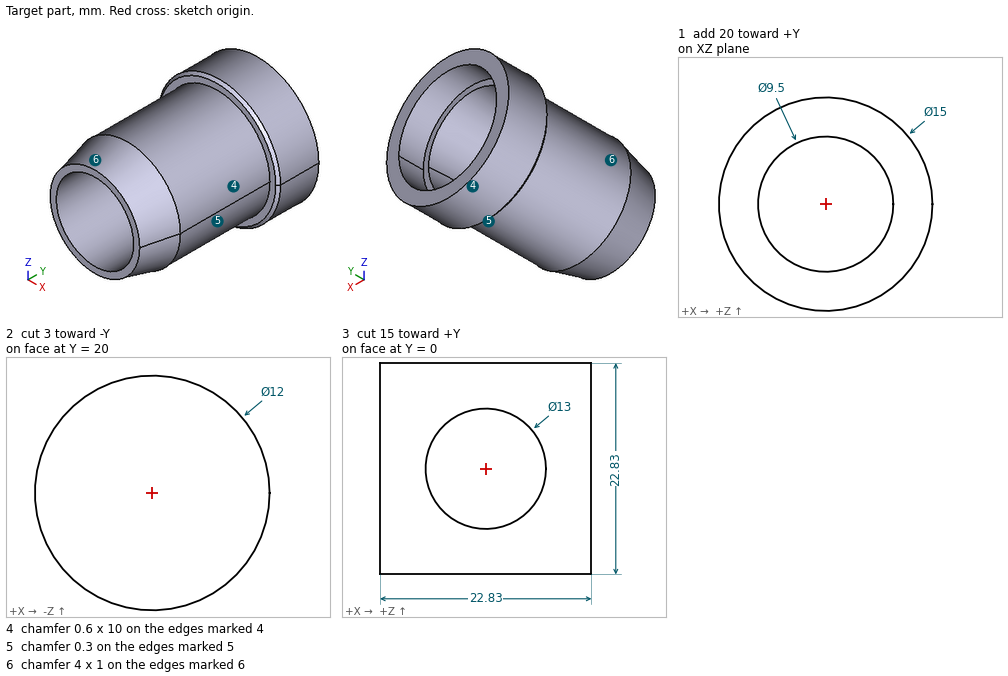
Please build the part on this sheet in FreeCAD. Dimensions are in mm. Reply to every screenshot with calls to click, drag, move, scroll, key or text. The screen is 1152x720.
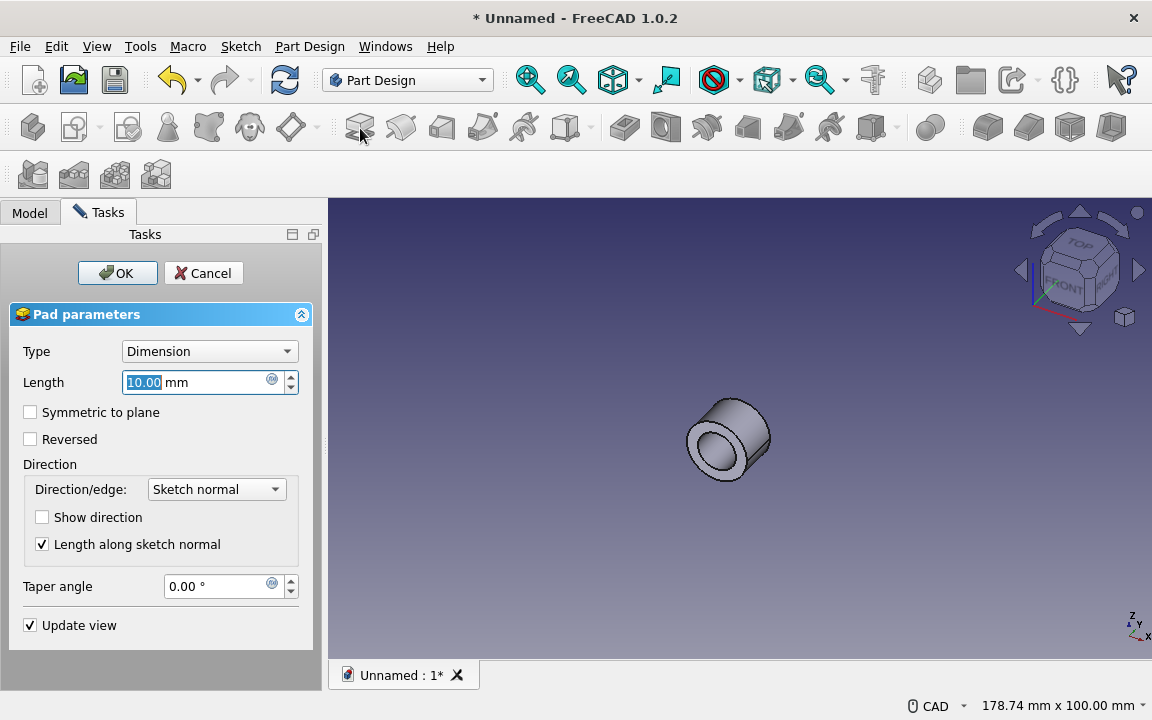
text(20)
key(Tab)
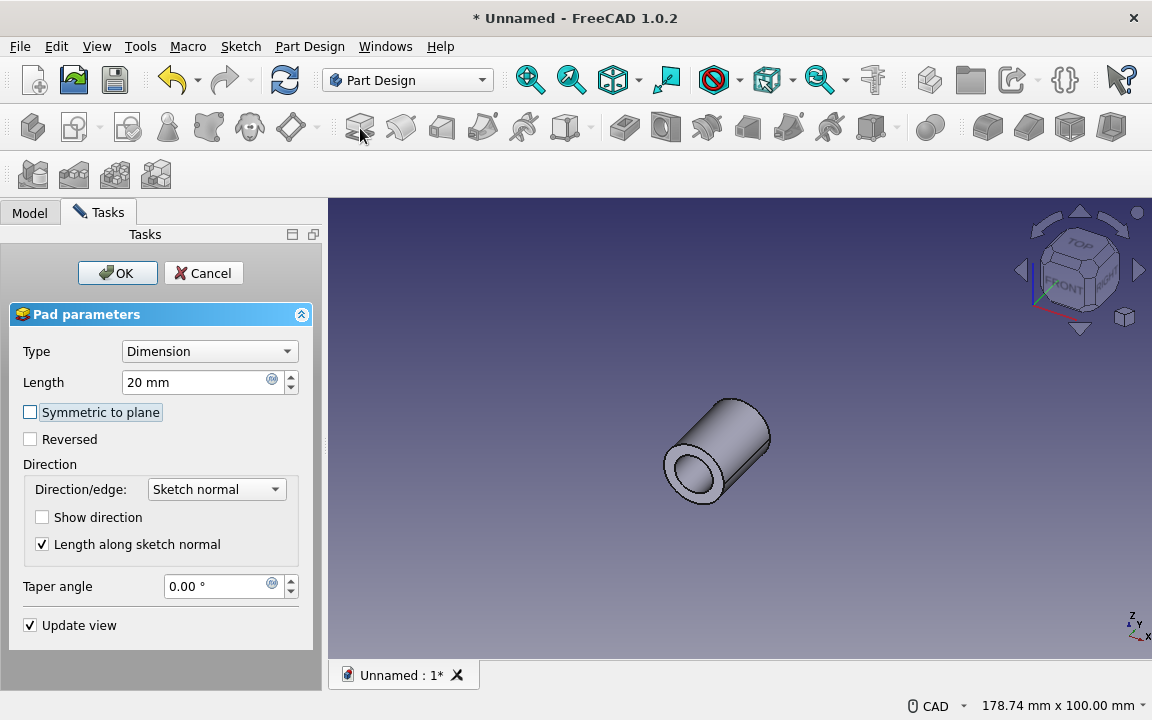
click(31, 439)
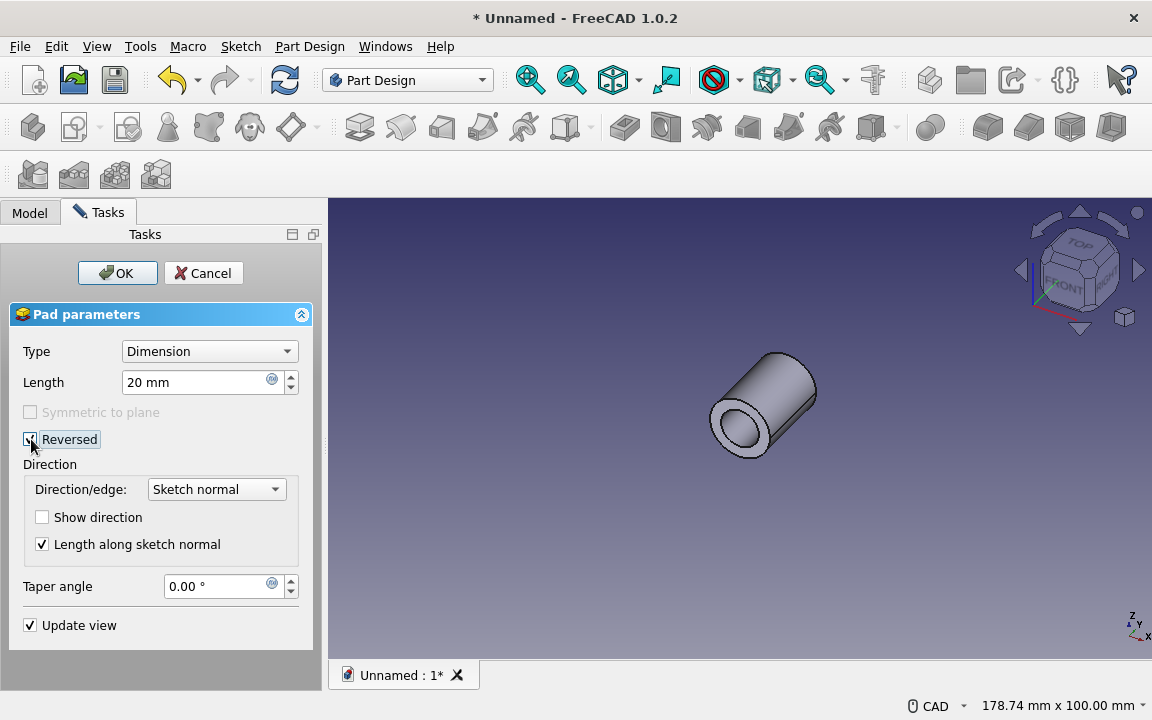
click(118, 273)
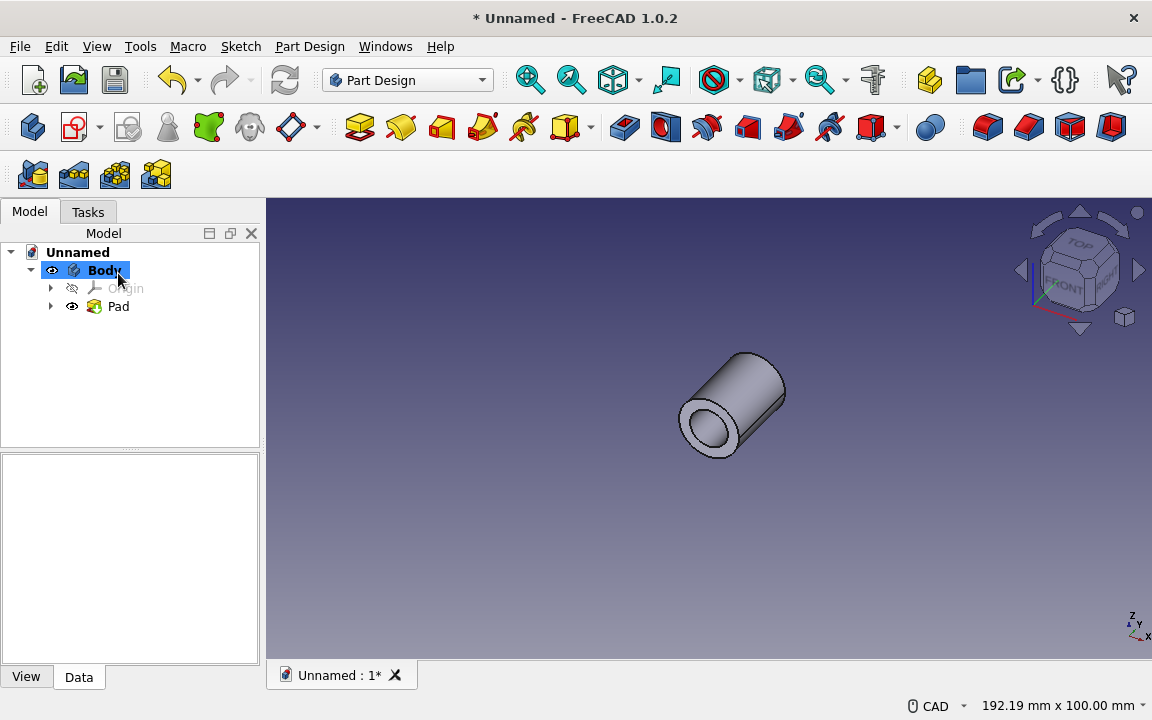
click(531, 80)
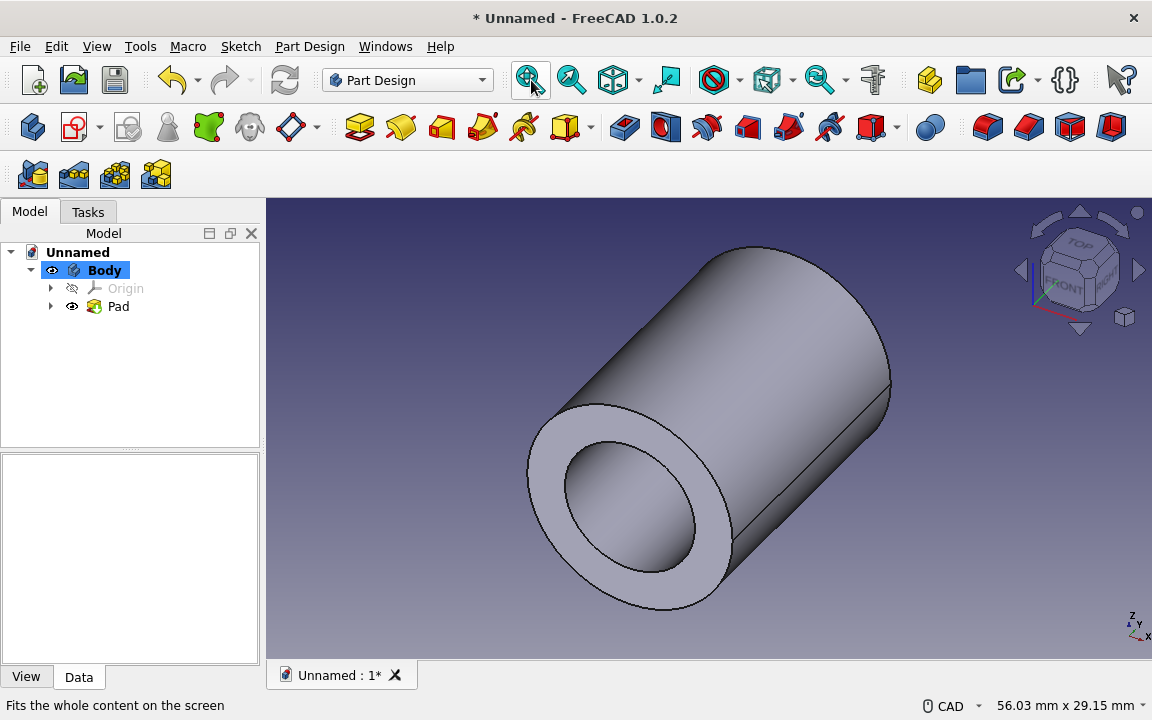
key(4)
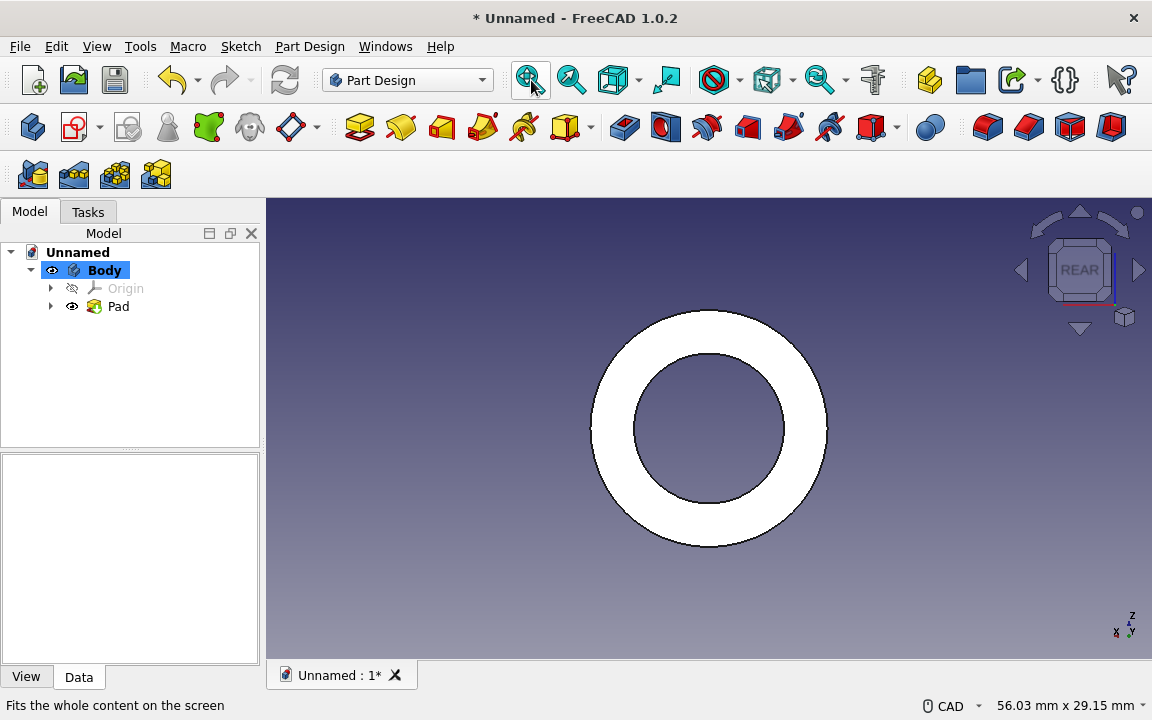
click(641, 360)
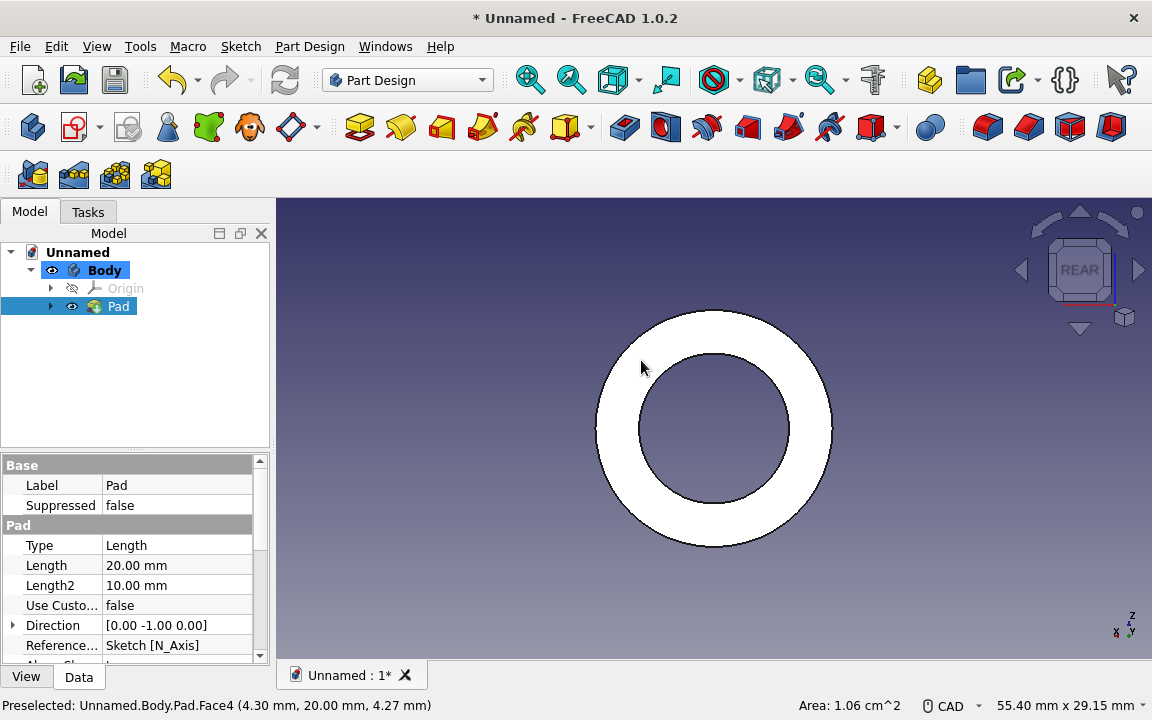
click(74, 128)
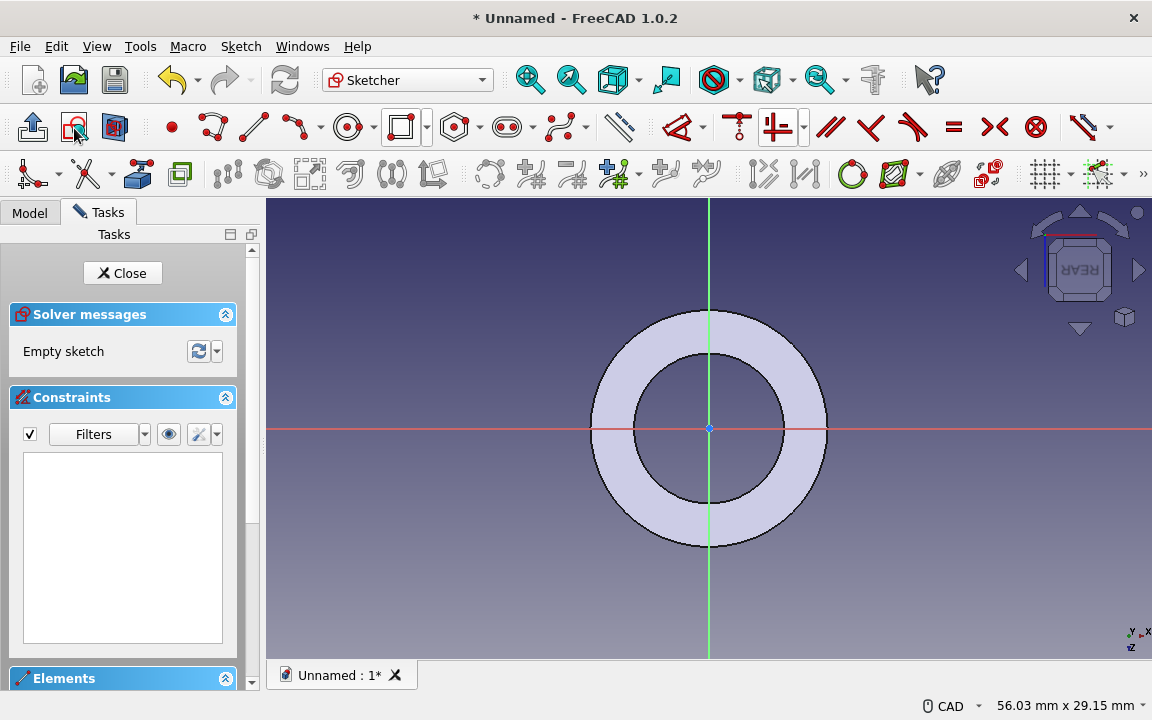
scroll(848, 428, up, 2)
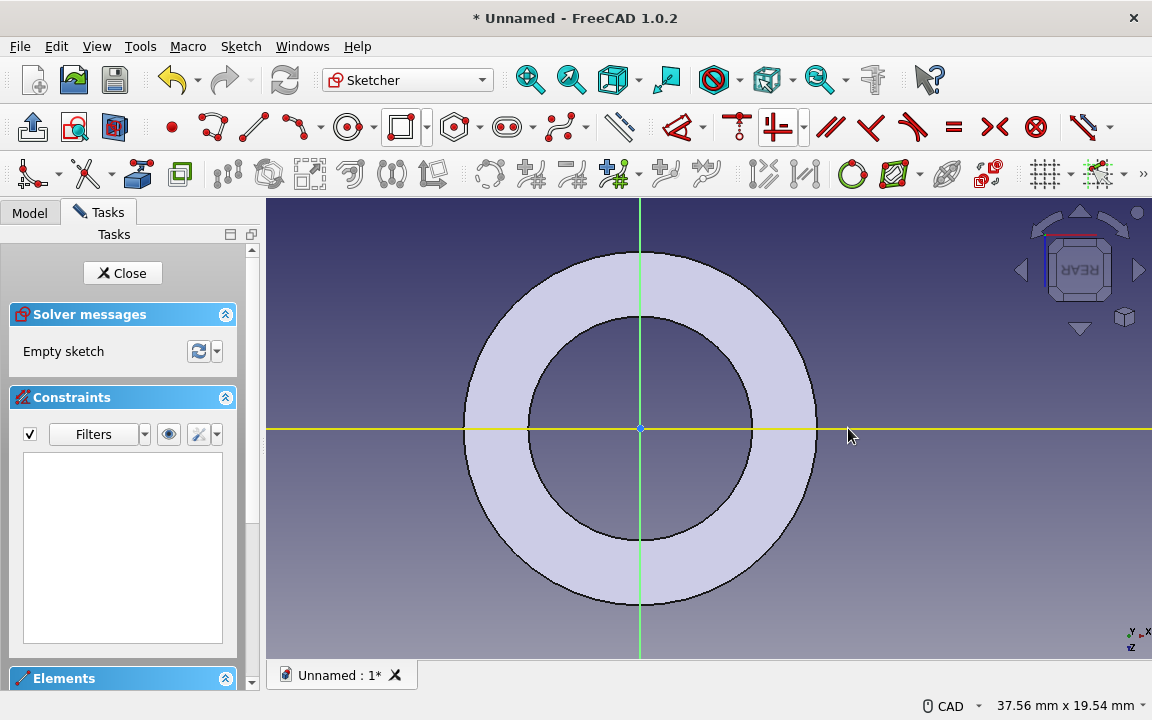
click(348, 128)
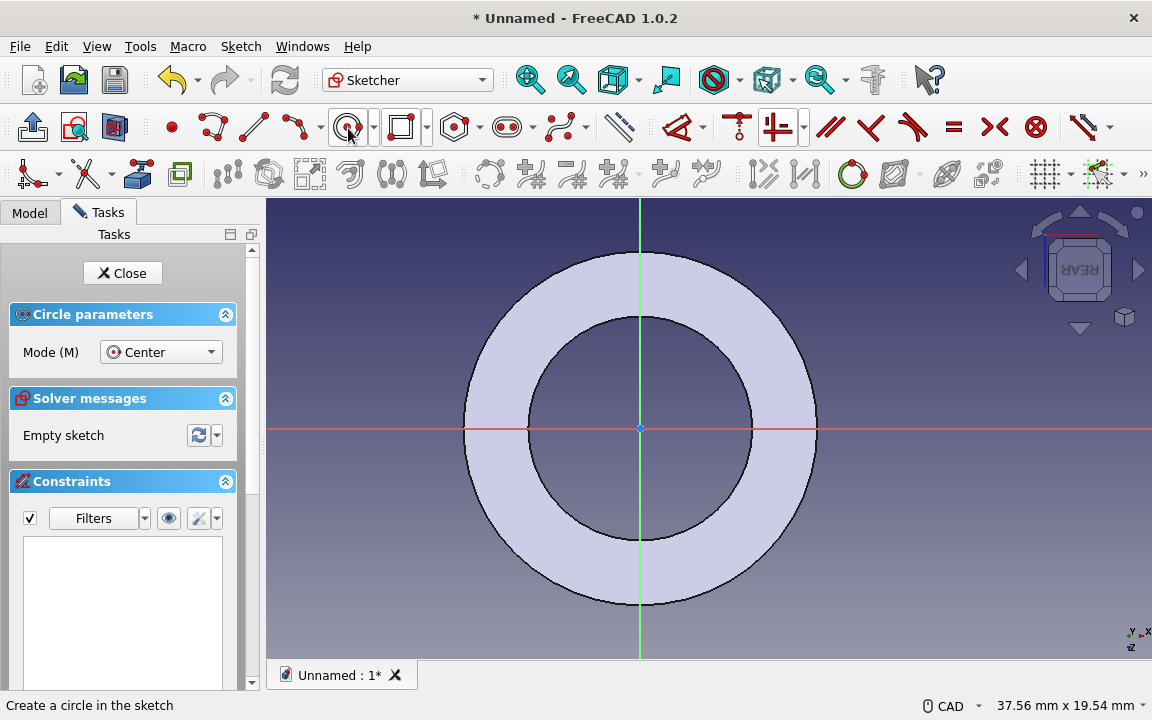
click(640, 428)
move(740, 328)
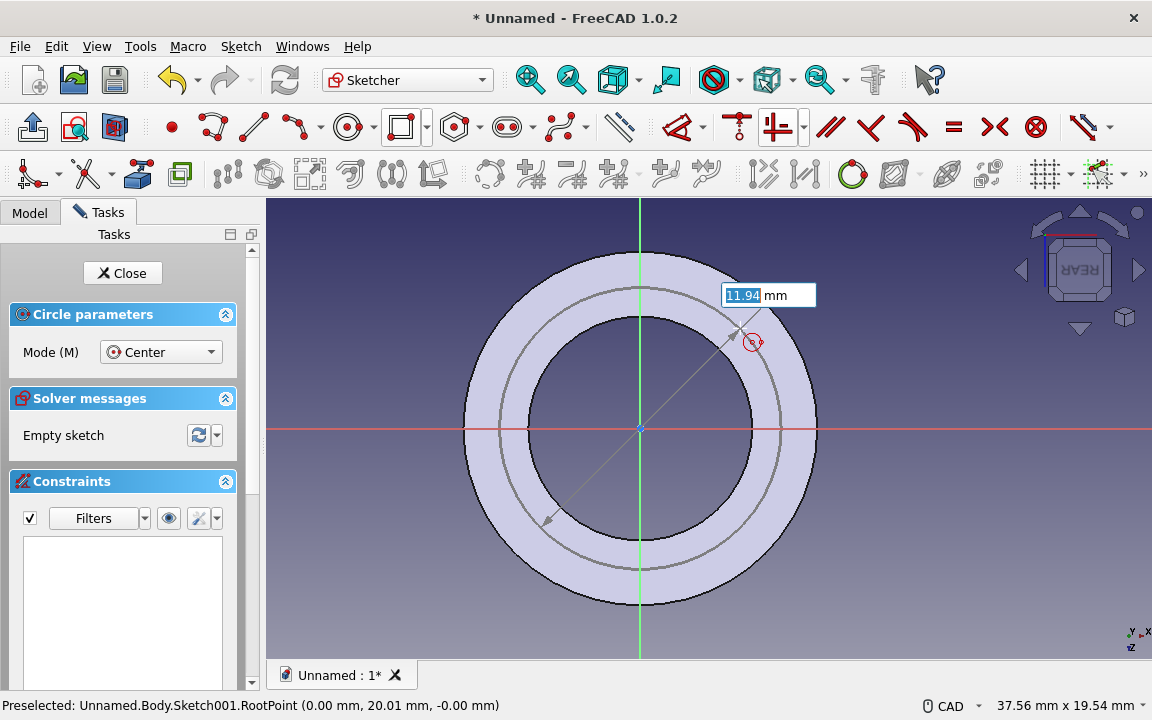
text(12)
key(Return)
key(Escape)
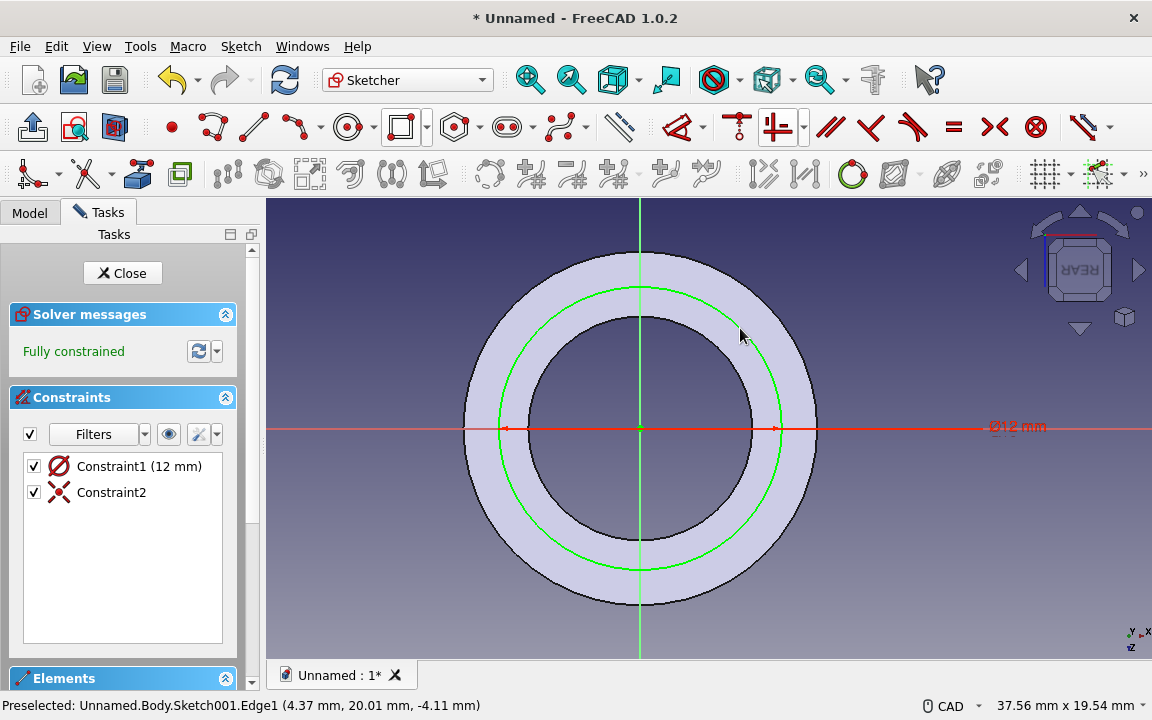
click(123, 273)